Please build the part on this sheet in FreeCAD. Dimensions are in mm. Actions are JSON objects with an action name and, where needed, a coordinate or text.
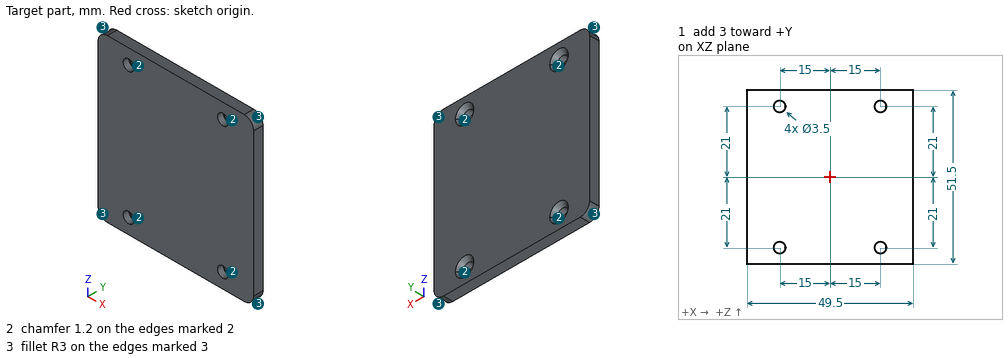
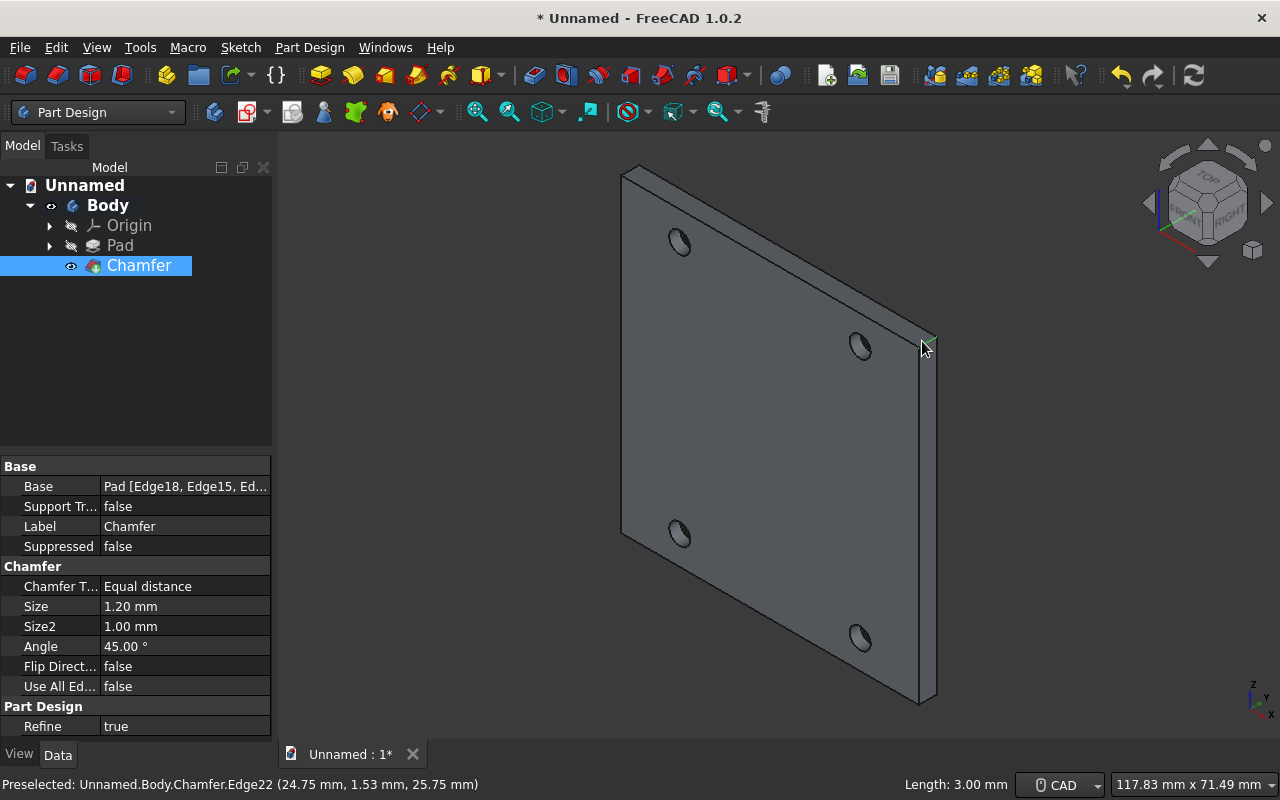
{"action": "key", "text": "2"}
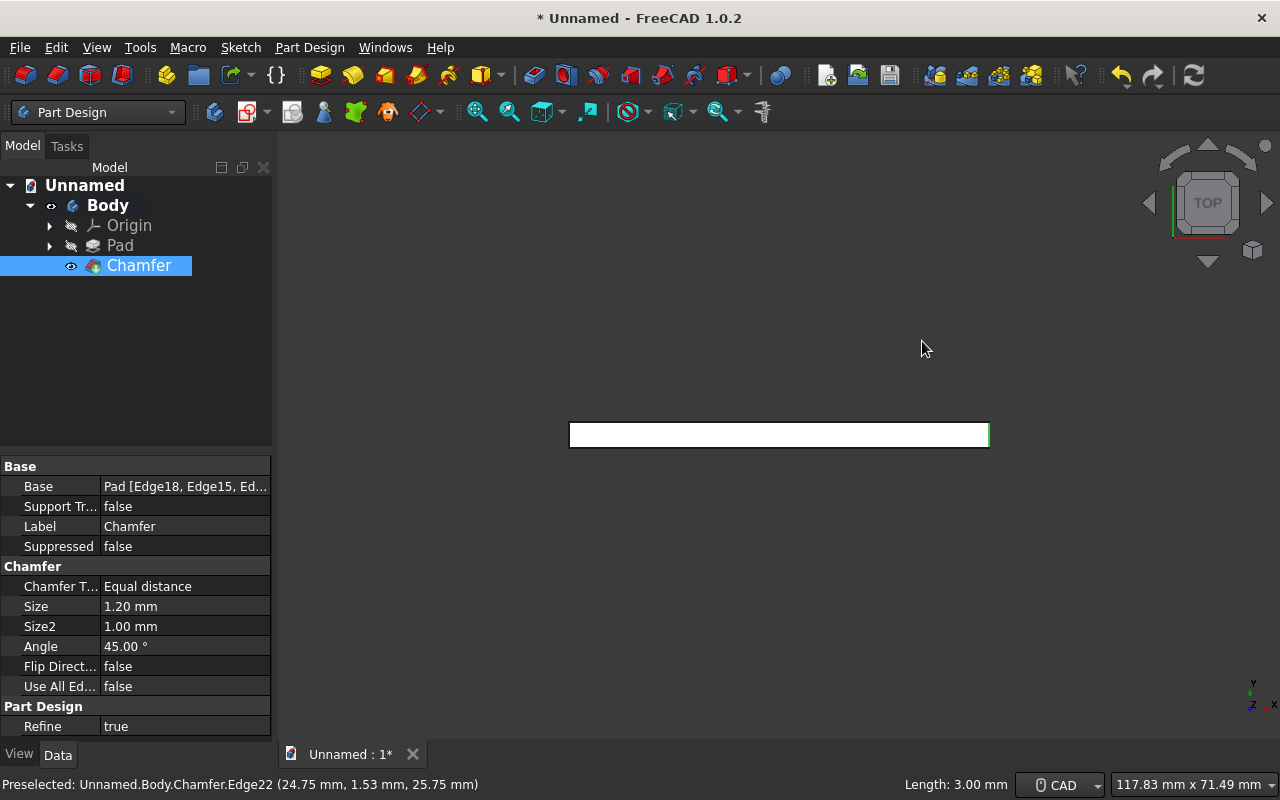
{"action": "left_click", "coordinate": [478, 112]}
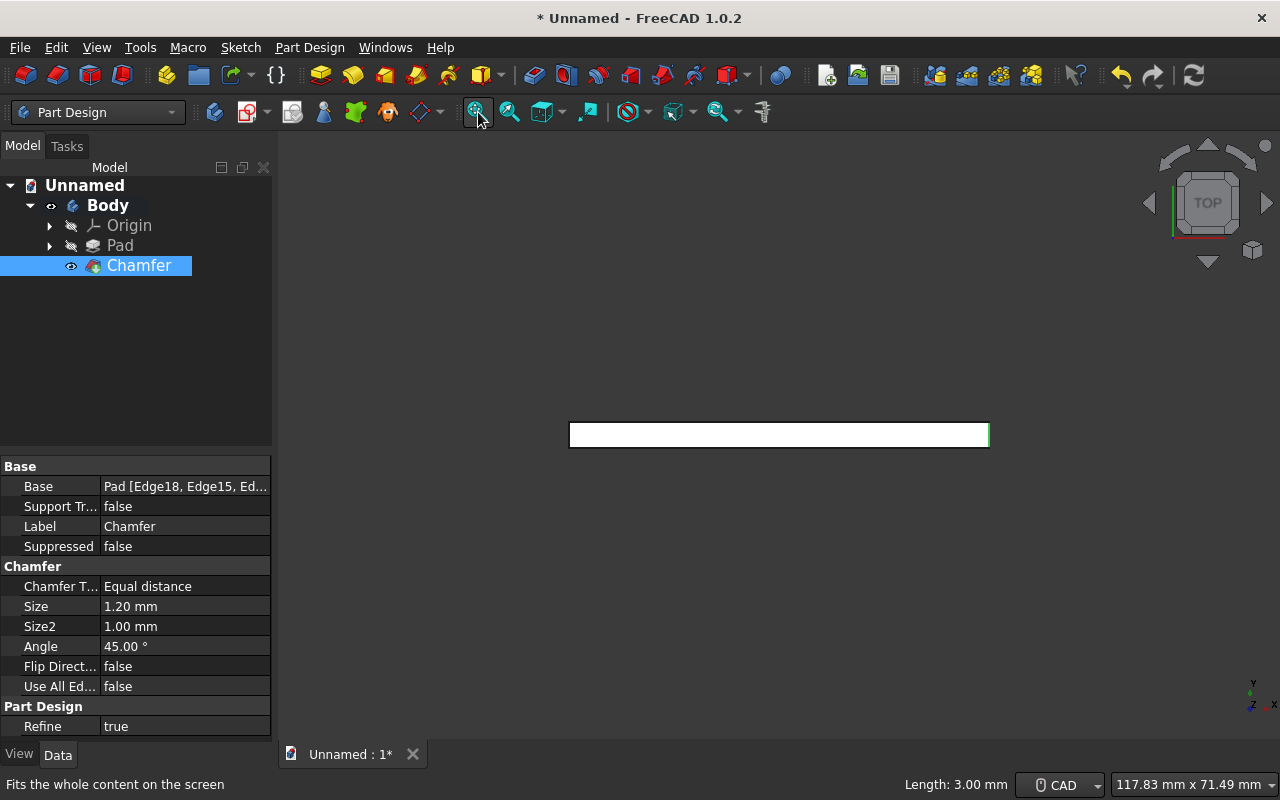
{"action": "left_click", "coordinate": [569, 434], "text": "ctrl"}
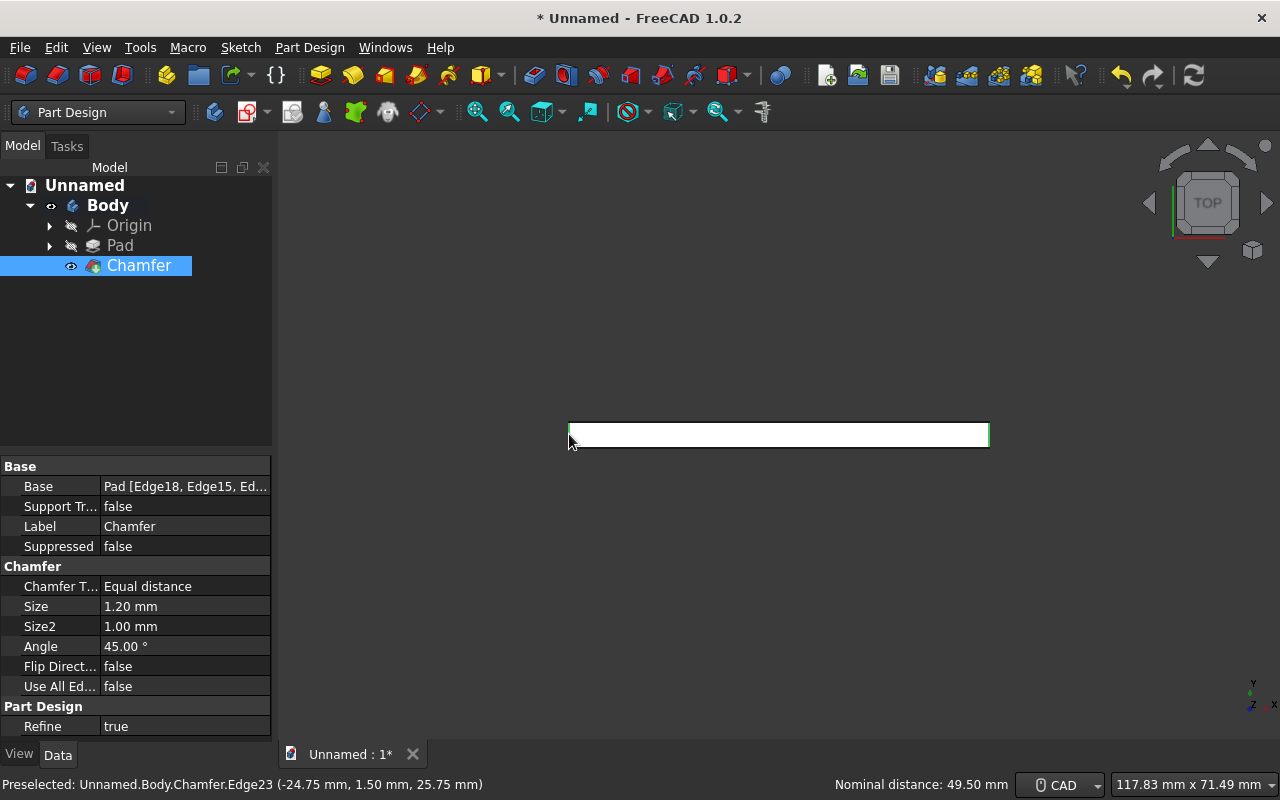
{"action": "key", "text": "1"}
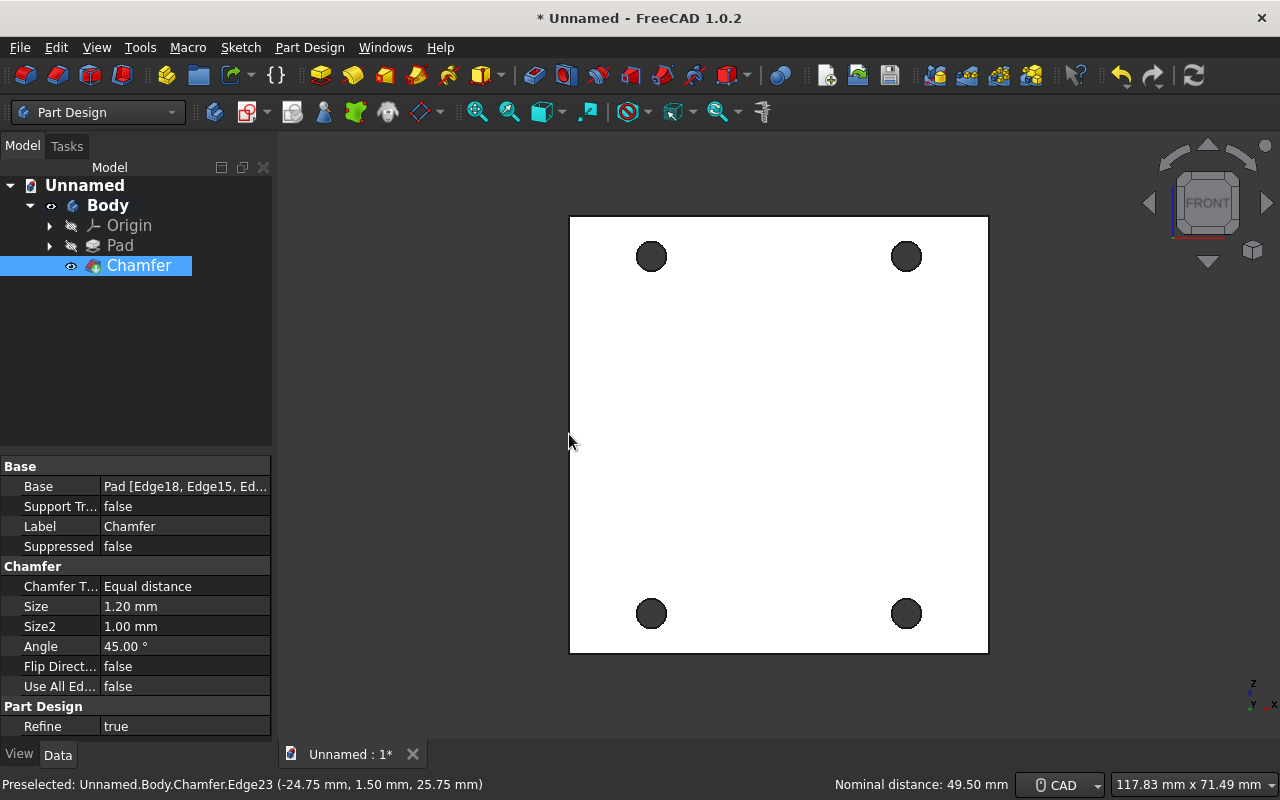
{"action": "key", "text": "3"}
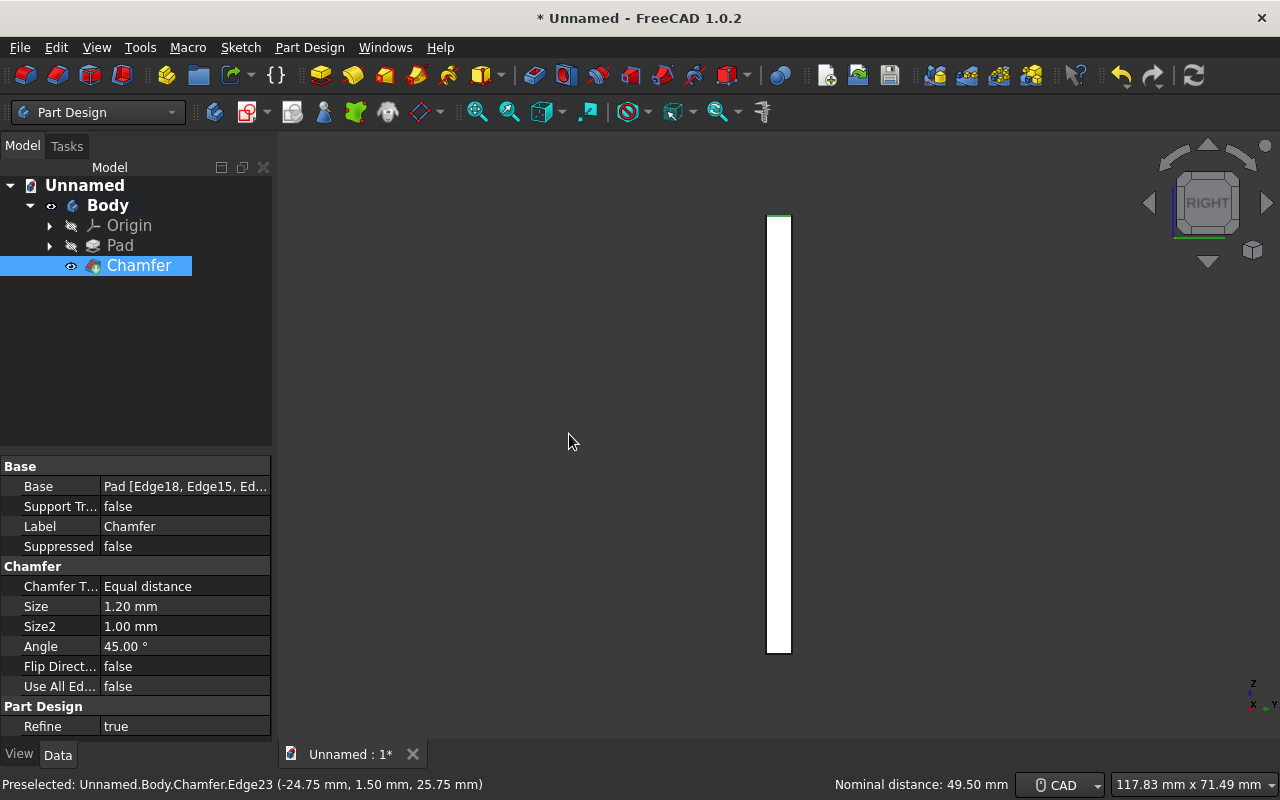
{"action": "left_click", "coordinate": [779, 653], "text": "ctrl"}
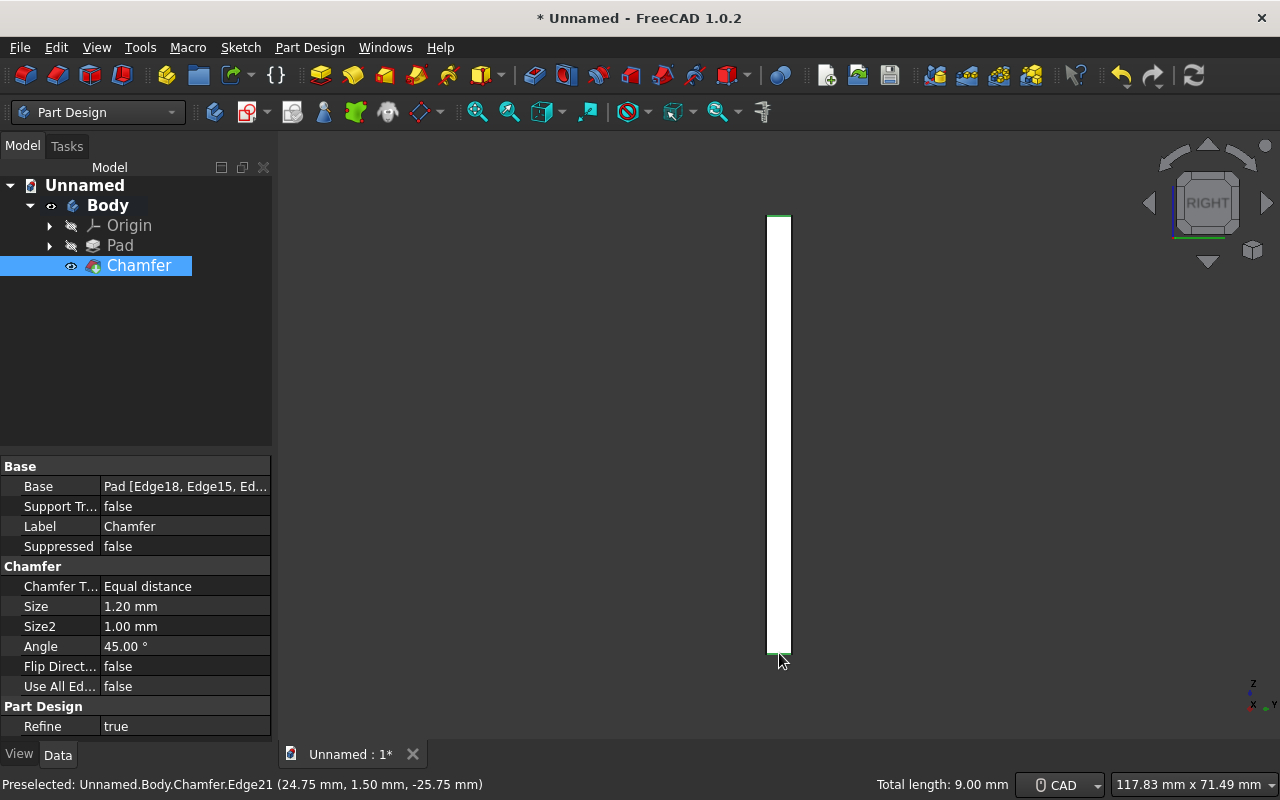
{"action": "key", "text": "5"}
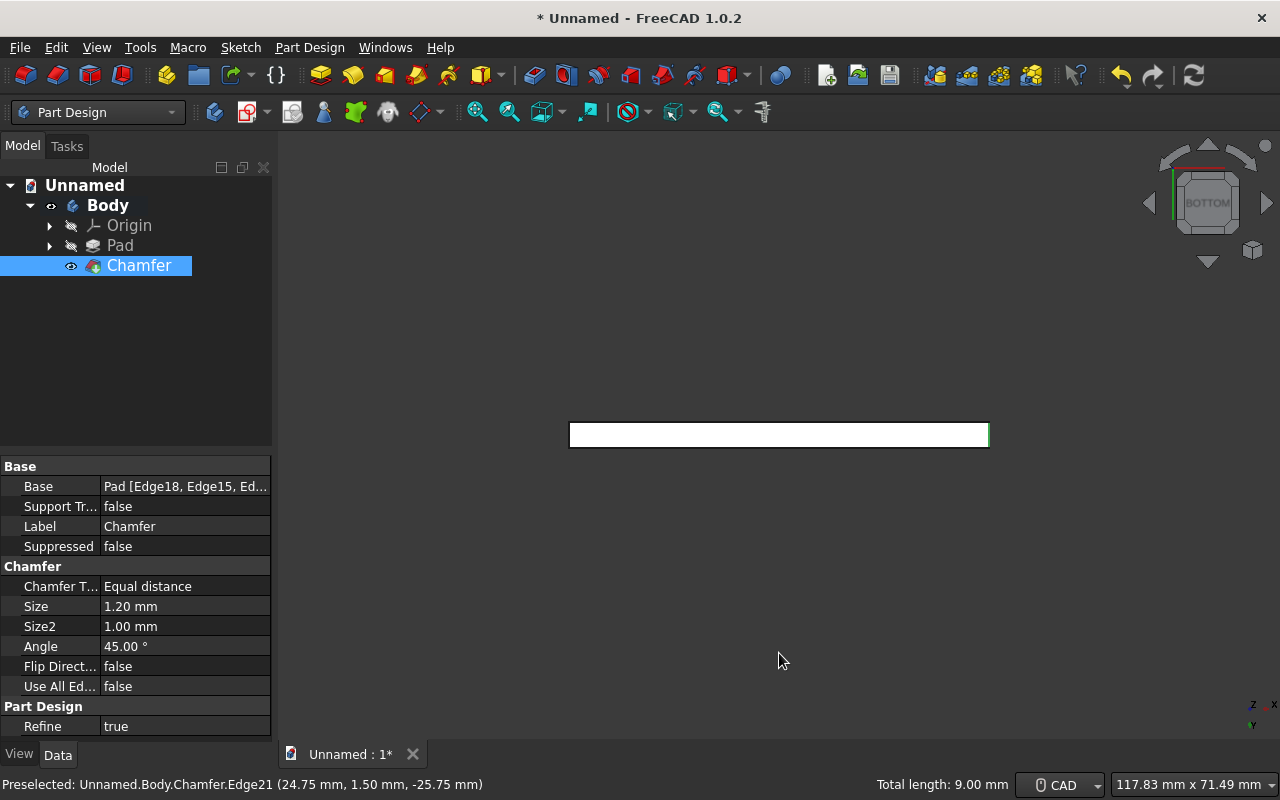
{"action": "left_click", "coordinate": [478, 112]}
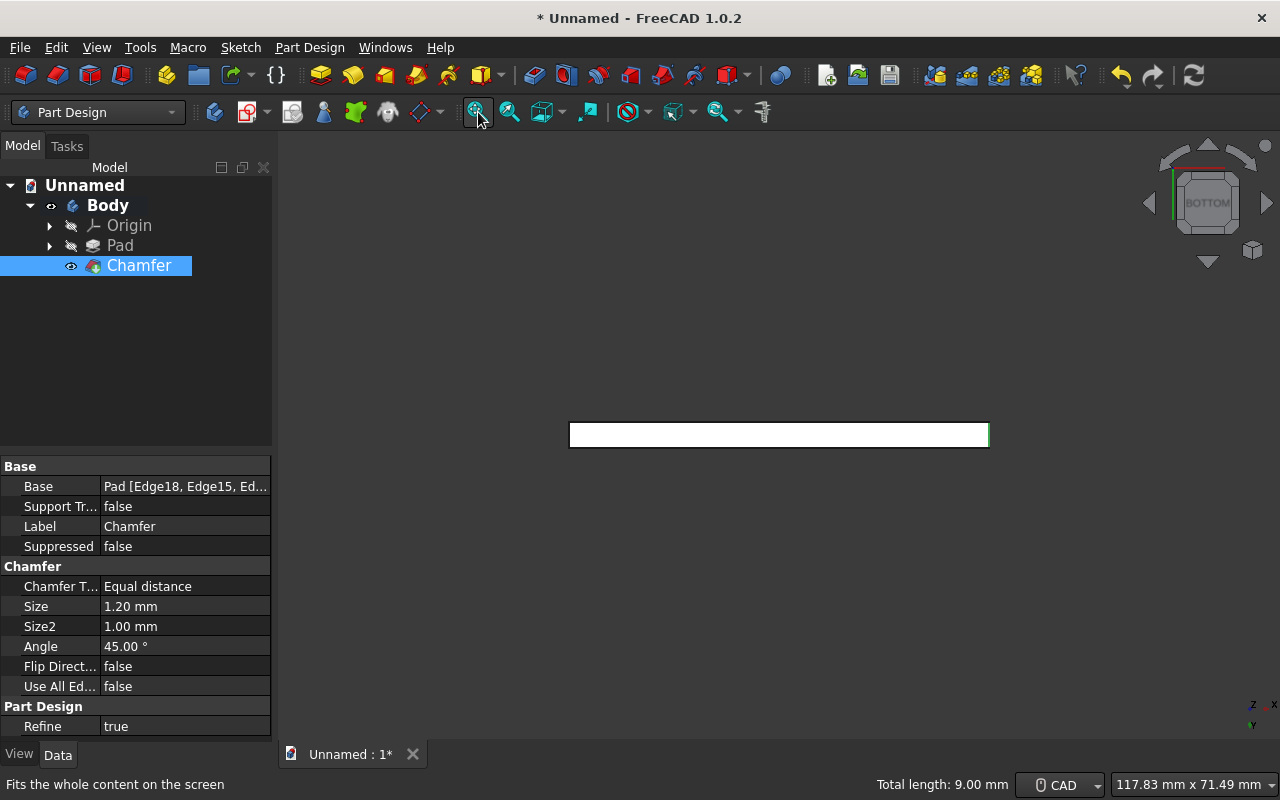
{"action": "left_click", "coordinate": [569, 434], "text": "ctrl"}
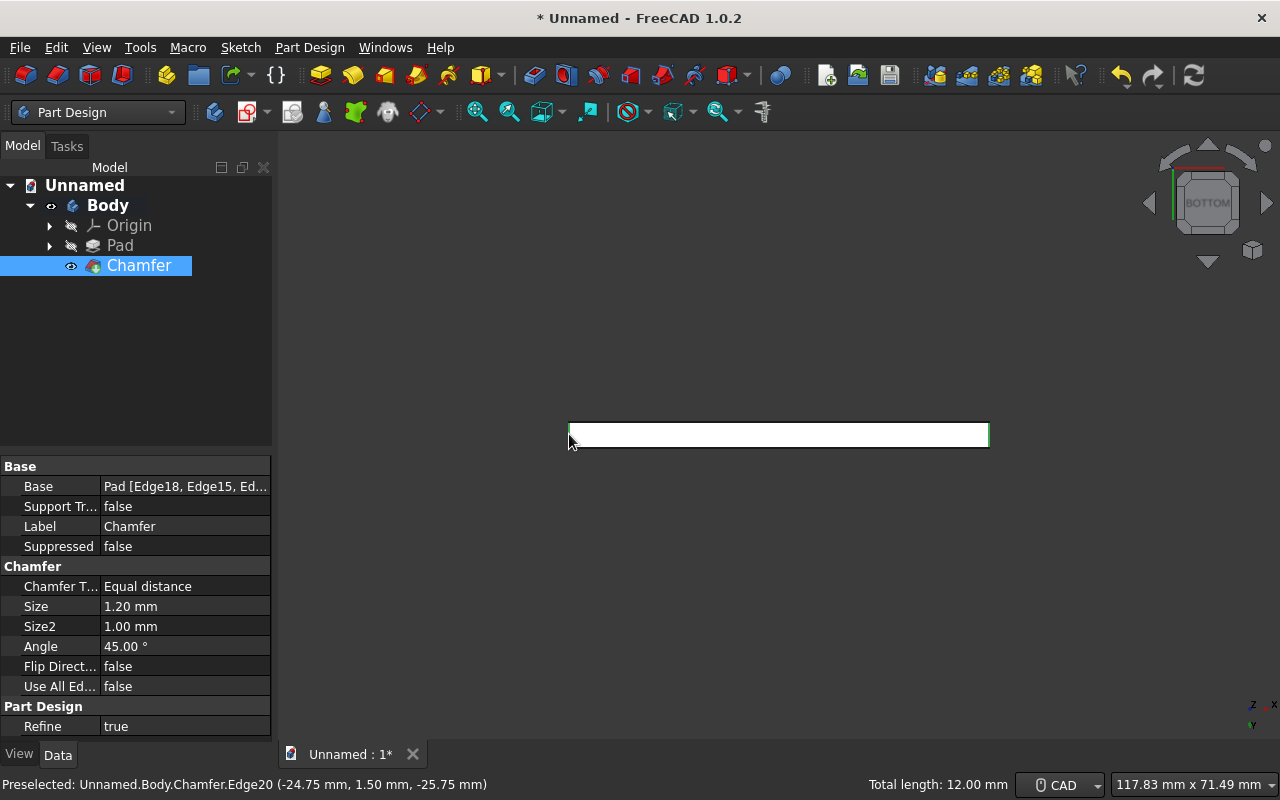
{"action": "left_click", "coordinate": [26, 76]}